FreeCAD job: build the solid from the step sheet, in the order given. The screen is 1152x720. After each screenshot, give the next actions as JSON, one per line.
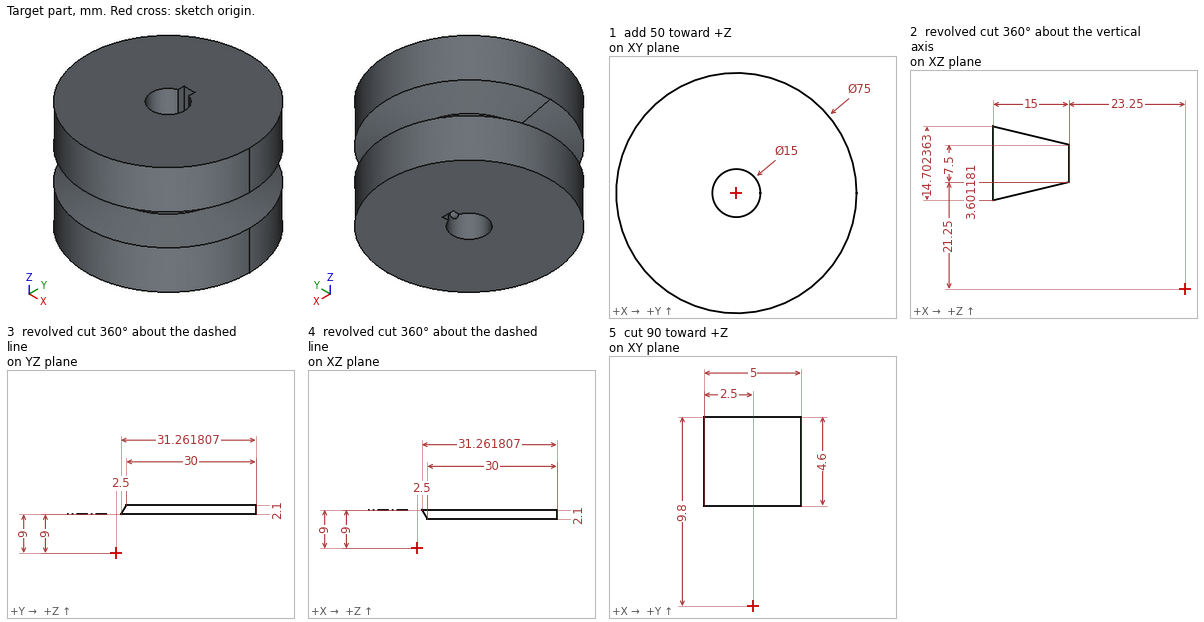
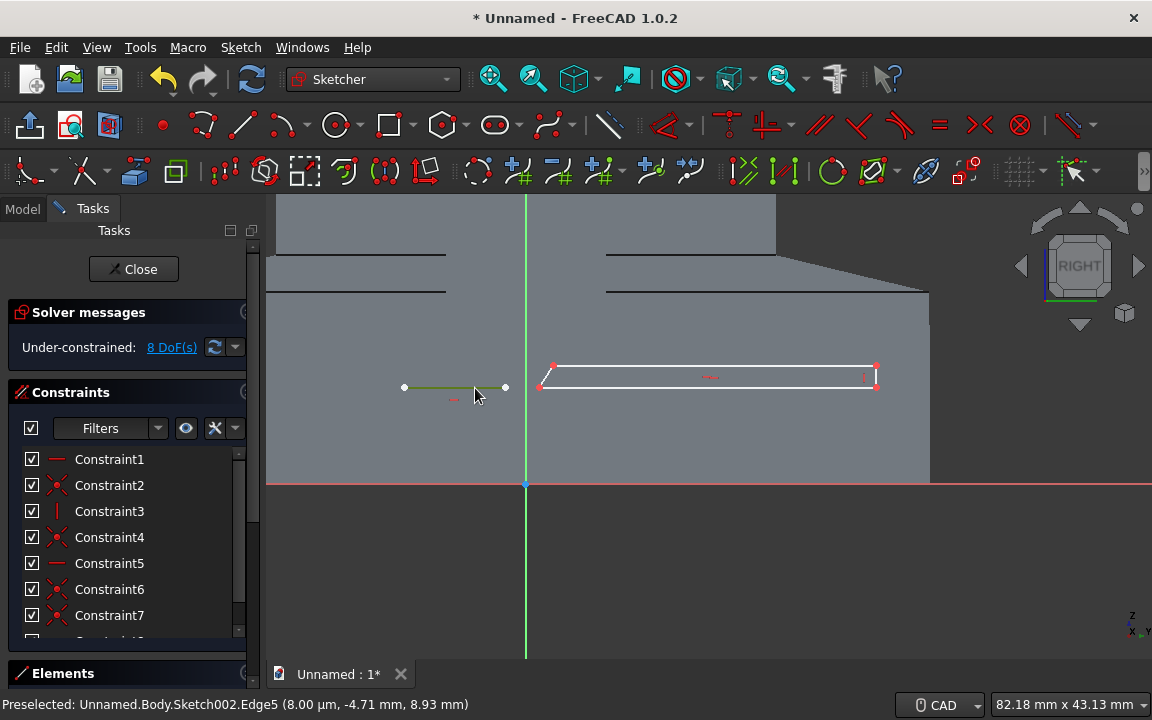
{"action": "key", "text": "g n"}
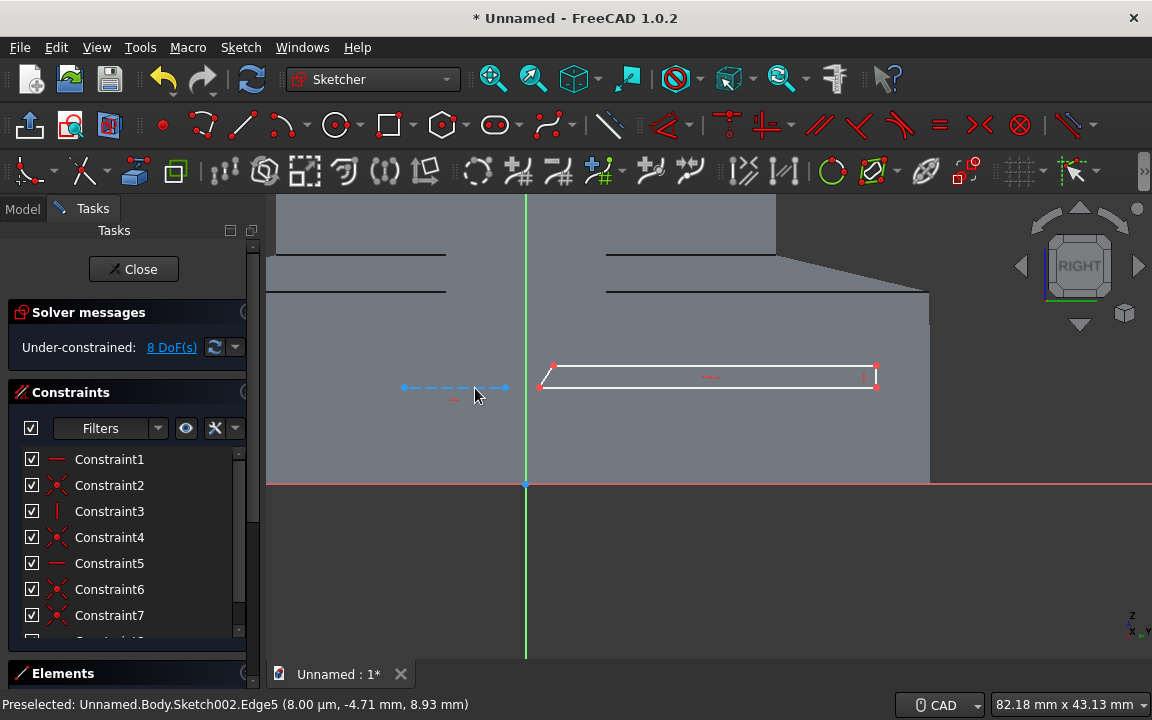
{"action": "left_click", "coordinate": [664, 126]}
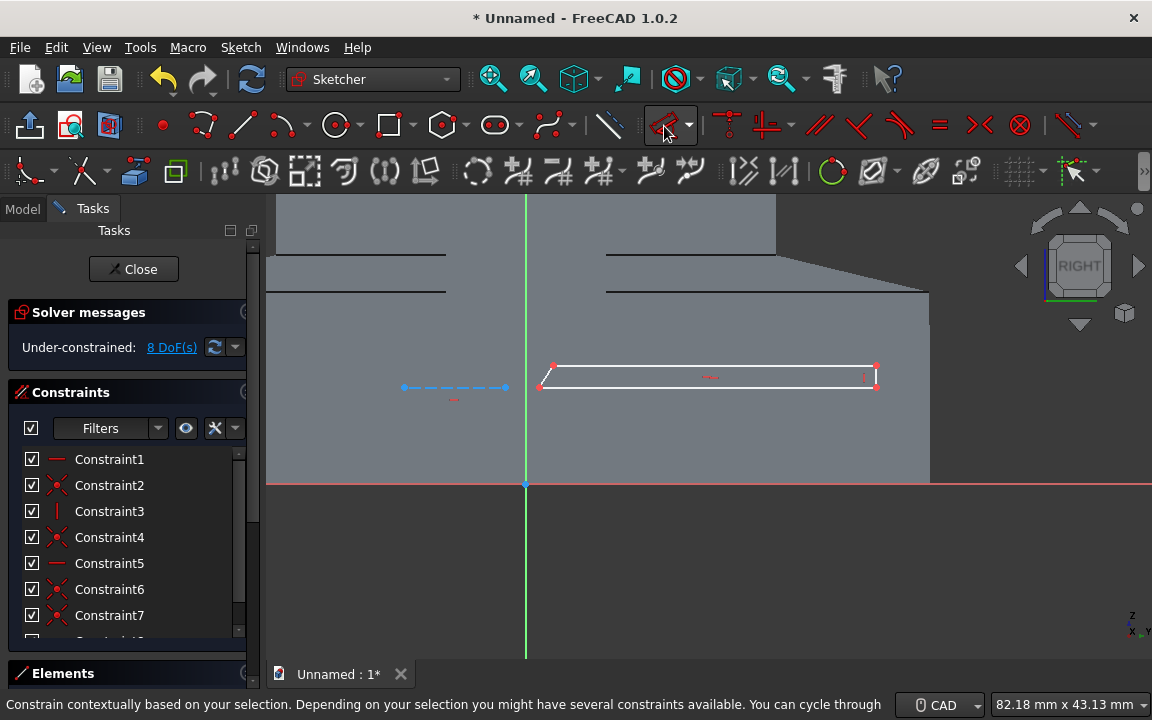
{"action": "left_click", "coordinate": [779, 366]}
{"action": "left_click", "coordinate": [715, 332]}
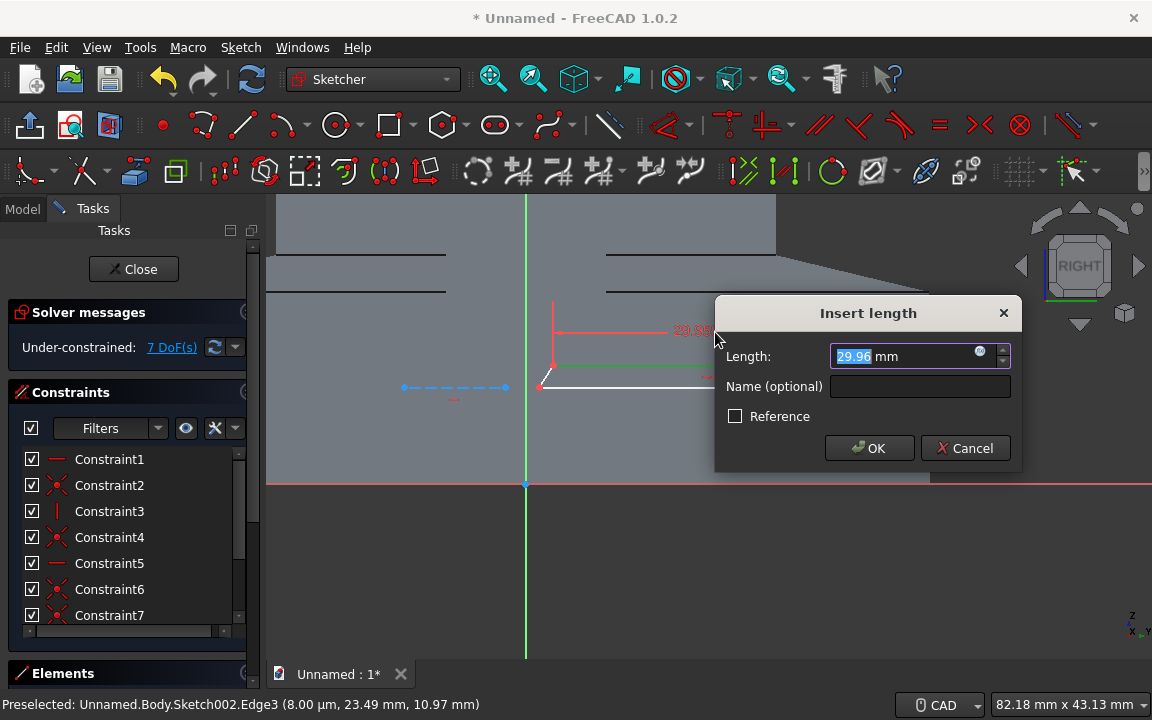
{"action": "type", "text": "30"}
{"action": "key", "text": "Return"}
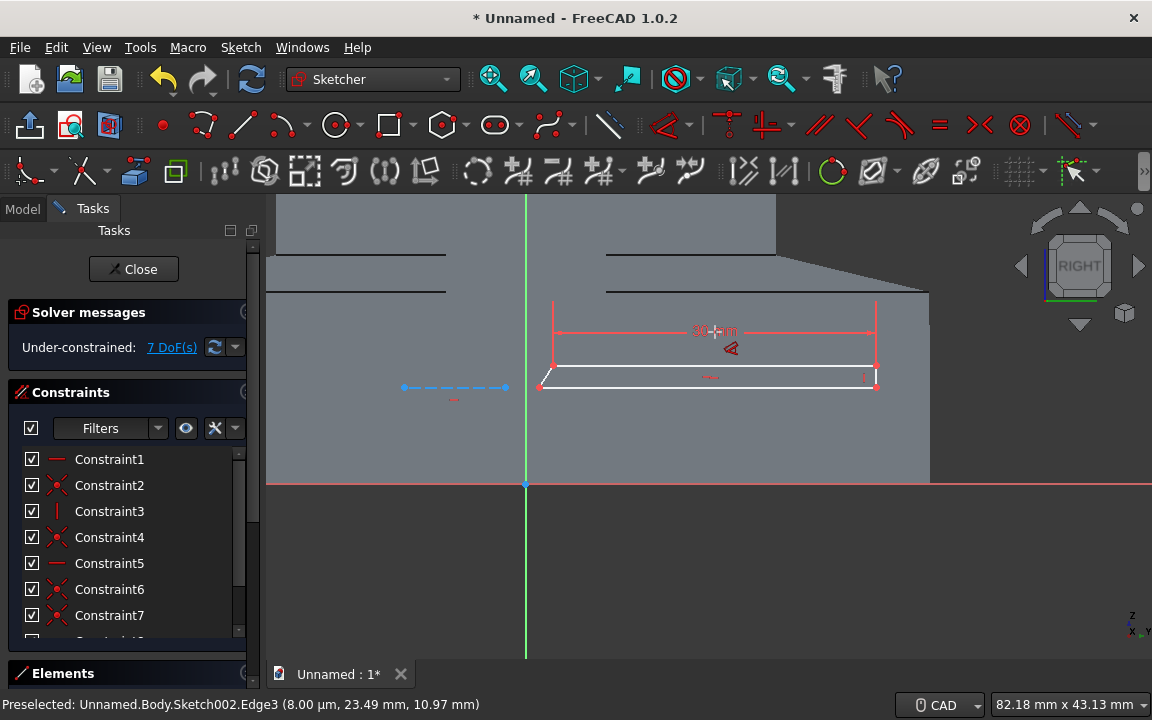
{"action": "left_click", "coordinate": [539, 388]}
{"action": "left_click", "coordinate": [492, 436]}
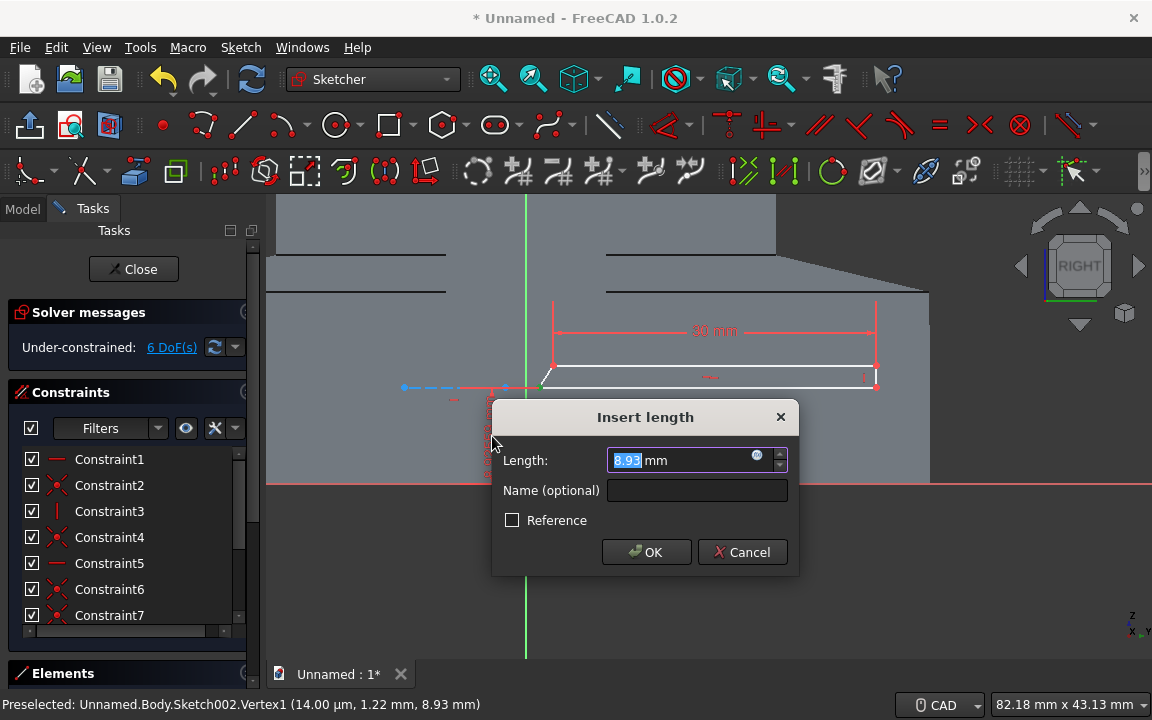
{"action": "type", "text": "9"}
{"action": "key", "text": "Return"}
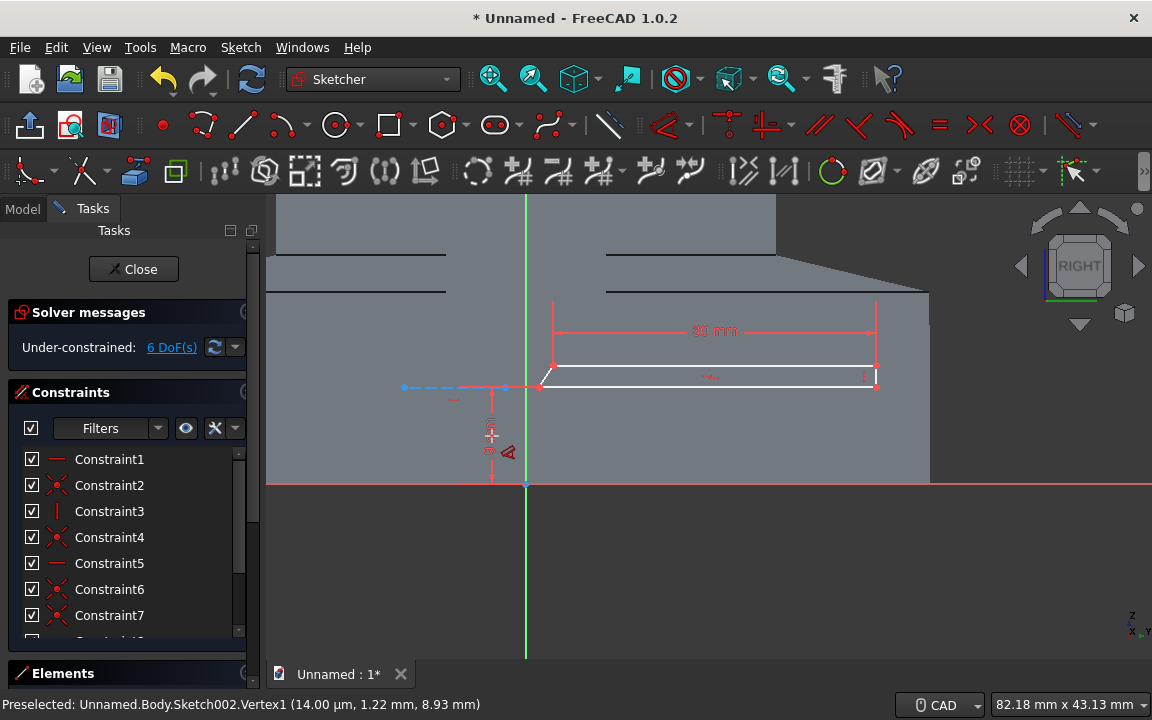
{"action": "left_click", "coordinate": [505, 388]}
{"action": "left_click", "coordinate": [471, 414]}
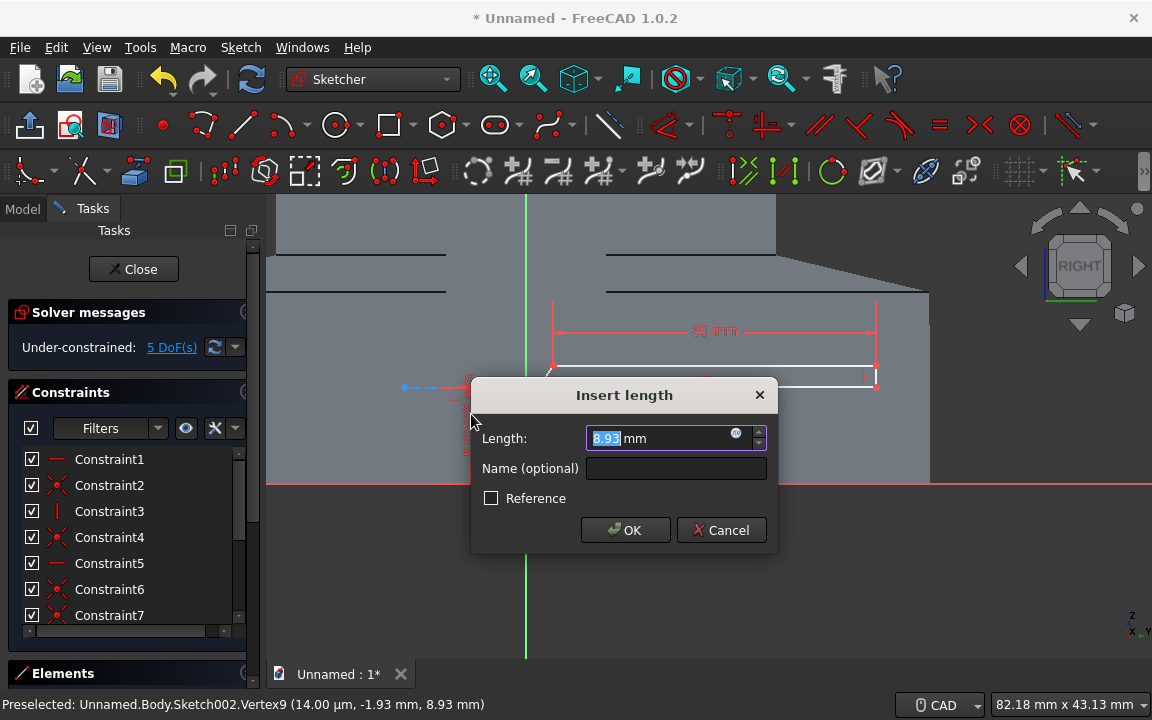
{"action": "type", "text": "9"}
{"action": "key", "text": "Return"}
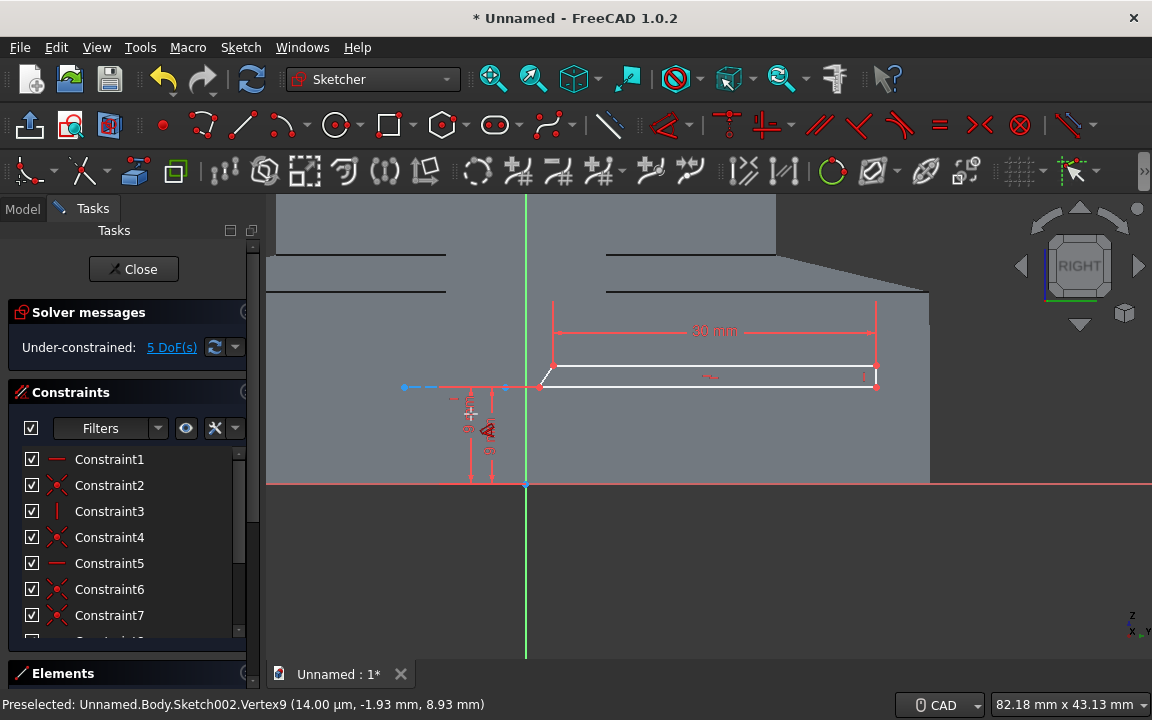
{"action": "scroll", "coordinate": [876, 377], "scroll_direction": "up", "scroll_amount": 3}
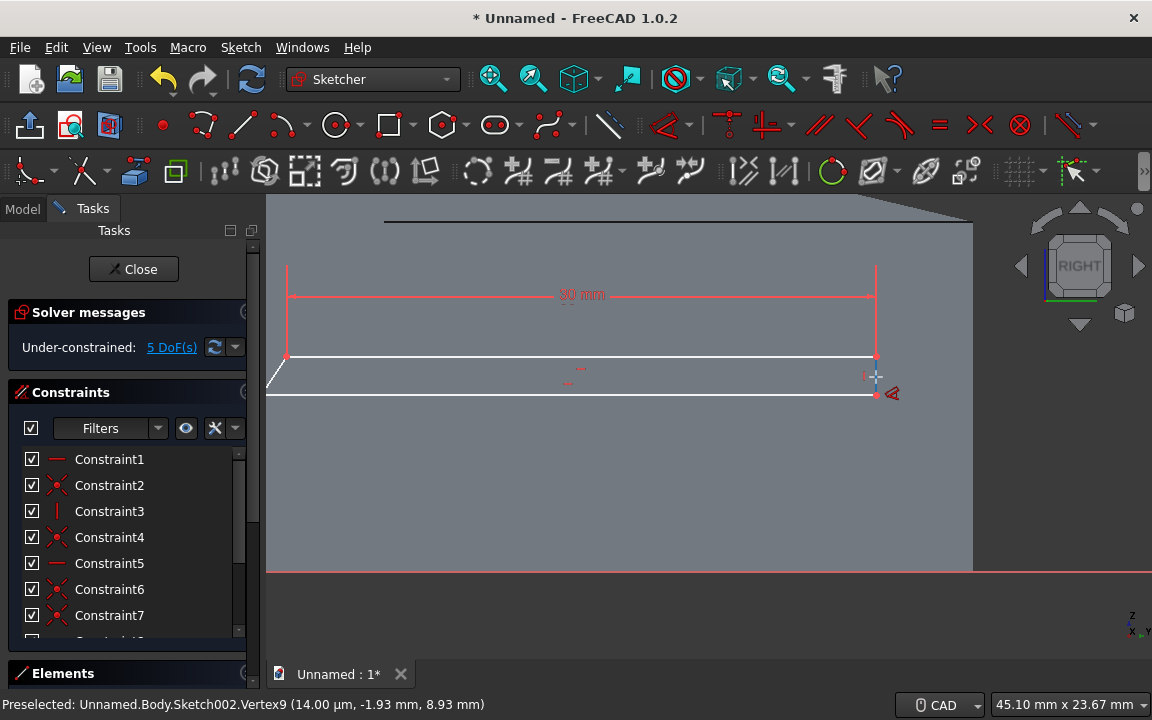
{"action": "left_click", "coordinate": [876, 376]}
{"action": "left_click", "coordinate": [910, 376]}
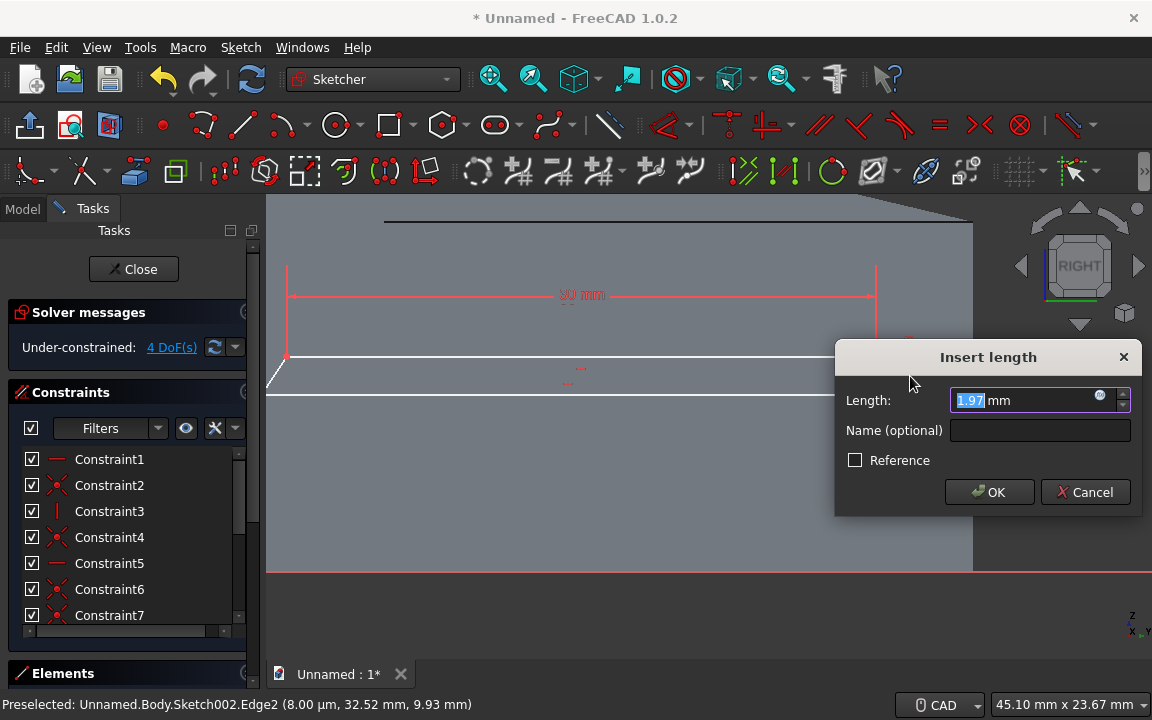
{"action": "type", "text": "2.1"}
{"action": "key", "text": "Return"}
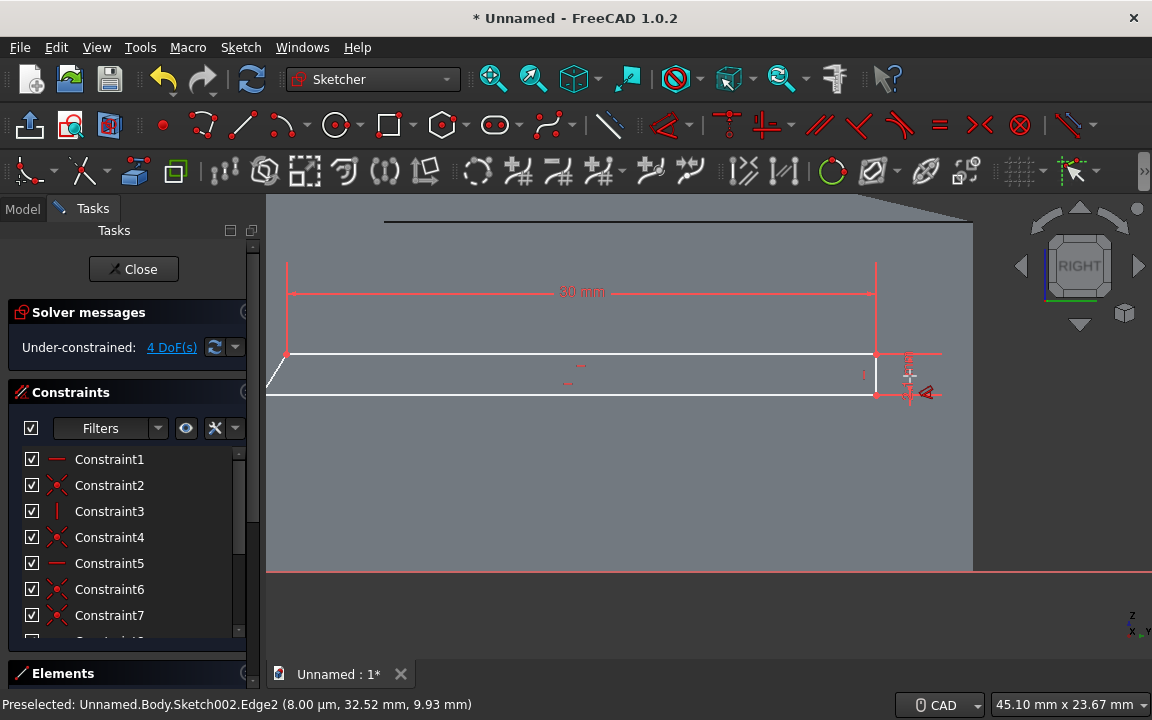
{"action": "scroll", "coordinate": [877, 382], "scroll_direction": "down", "scroll_amount": 3}